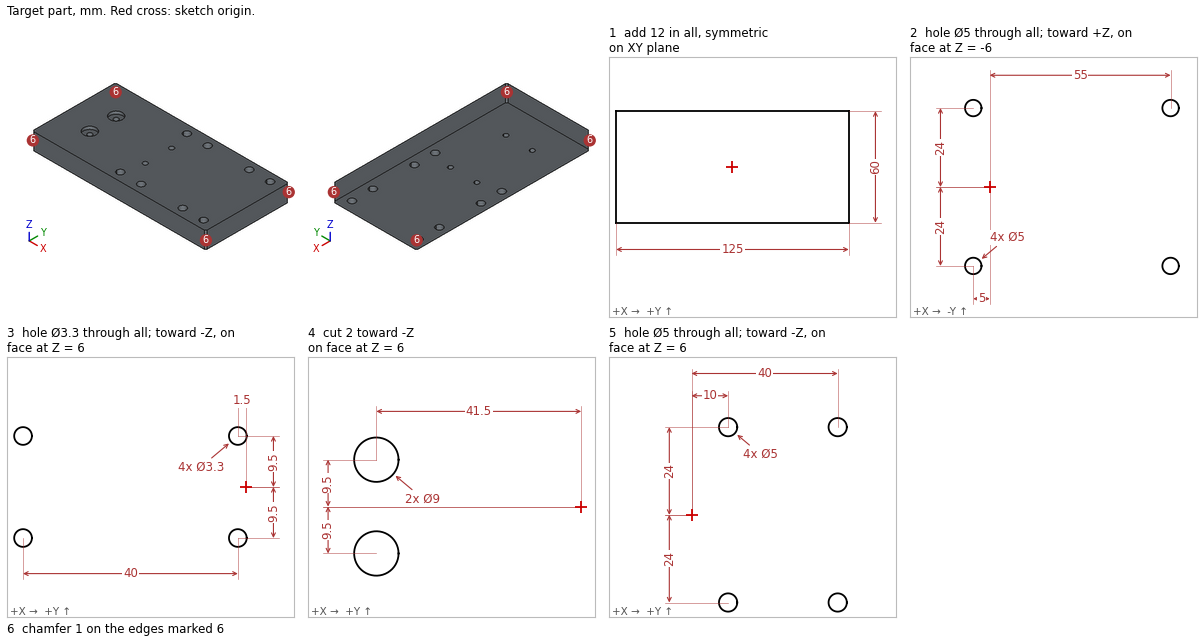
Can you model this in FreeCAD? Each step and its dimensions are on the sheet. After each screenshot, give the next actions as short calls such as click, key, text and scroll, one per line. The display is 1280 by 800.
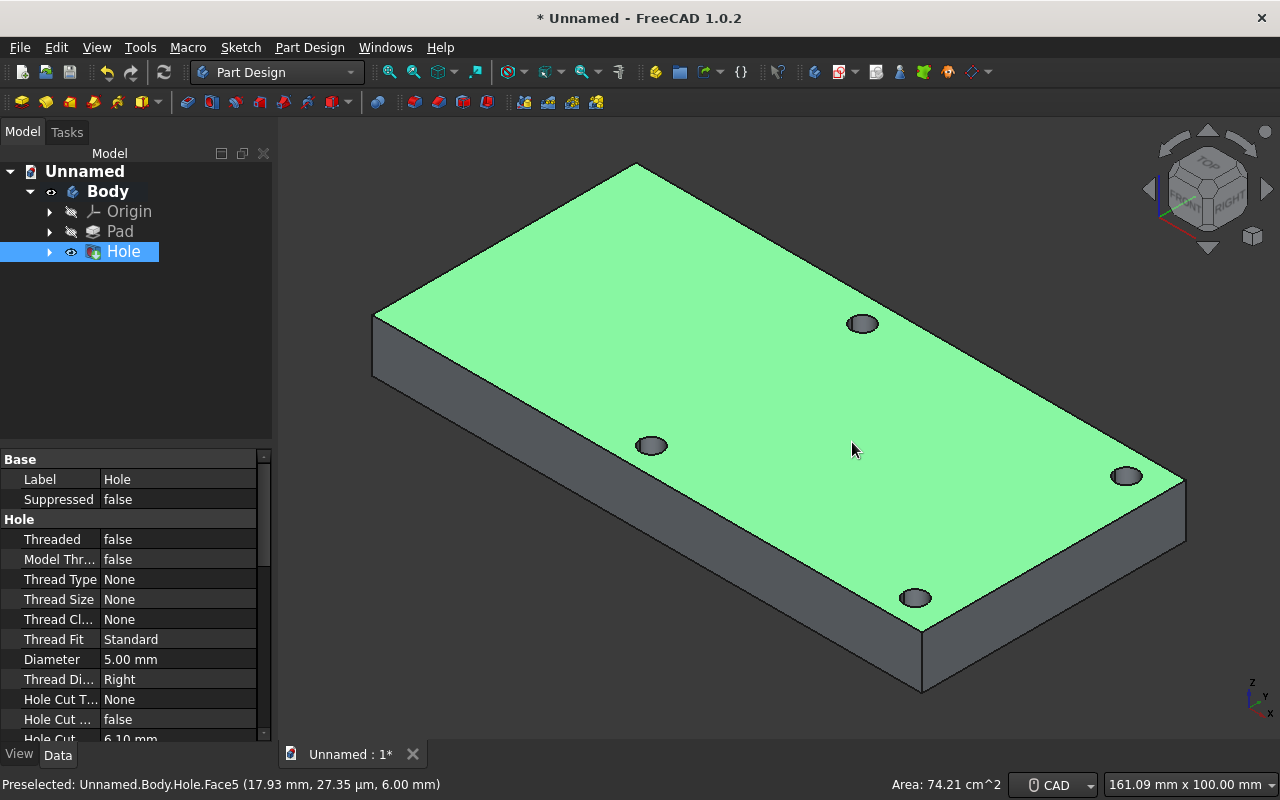
click(840, 72)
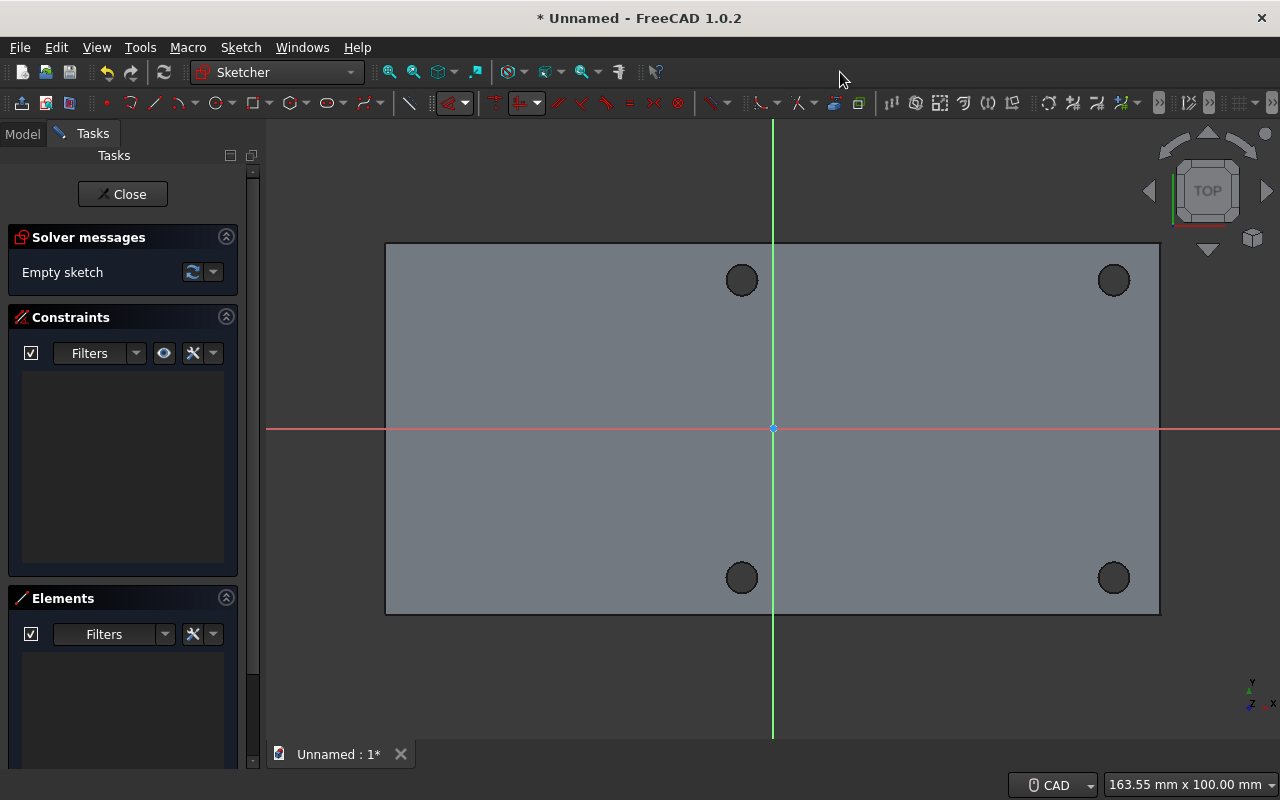
scroll(587, 429, up, 4)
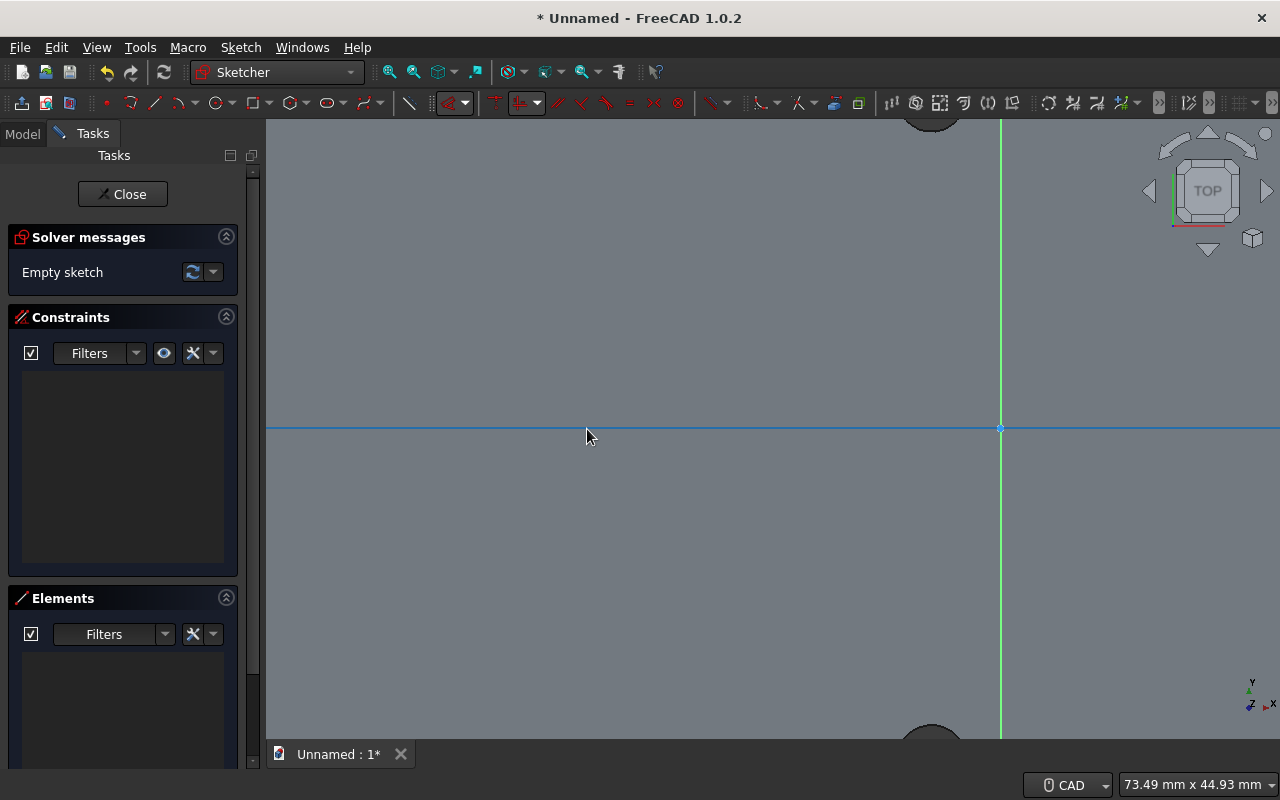
click(216, 104)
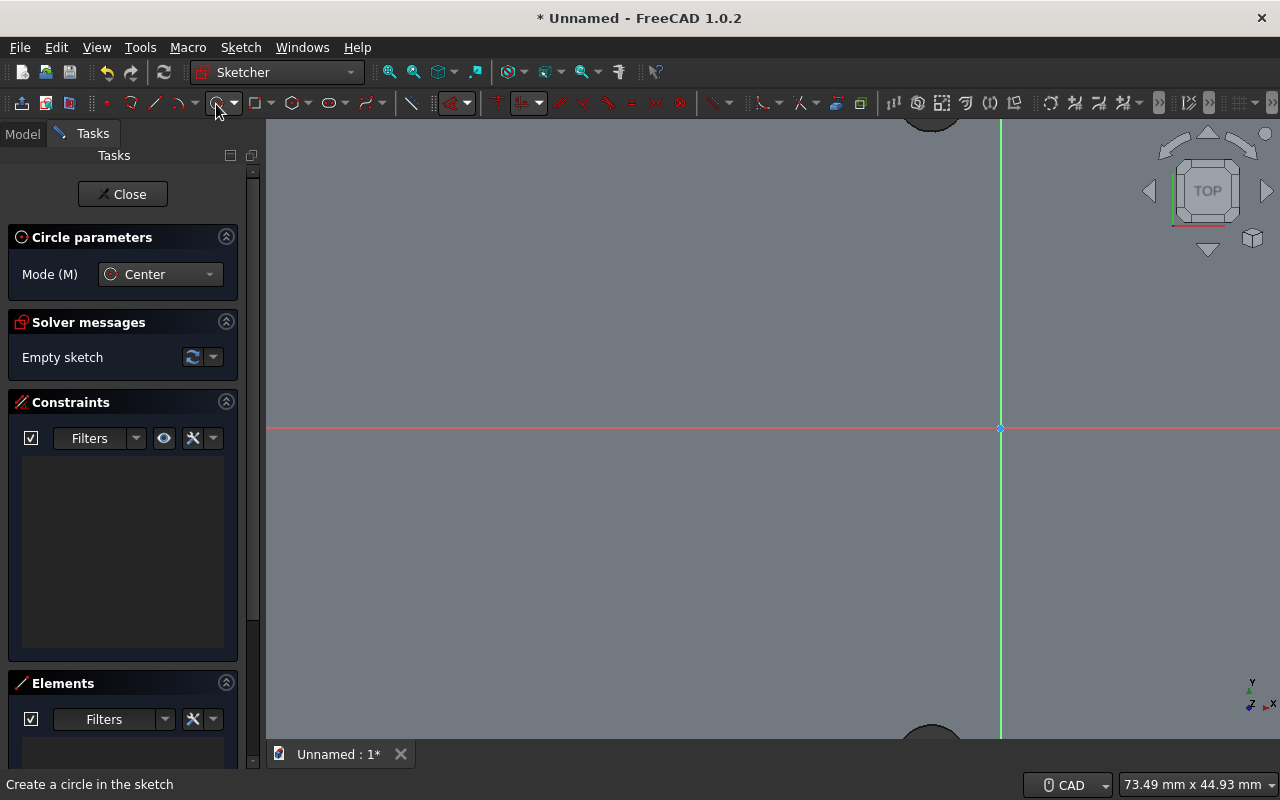
click(980, 297)
click(964, 281)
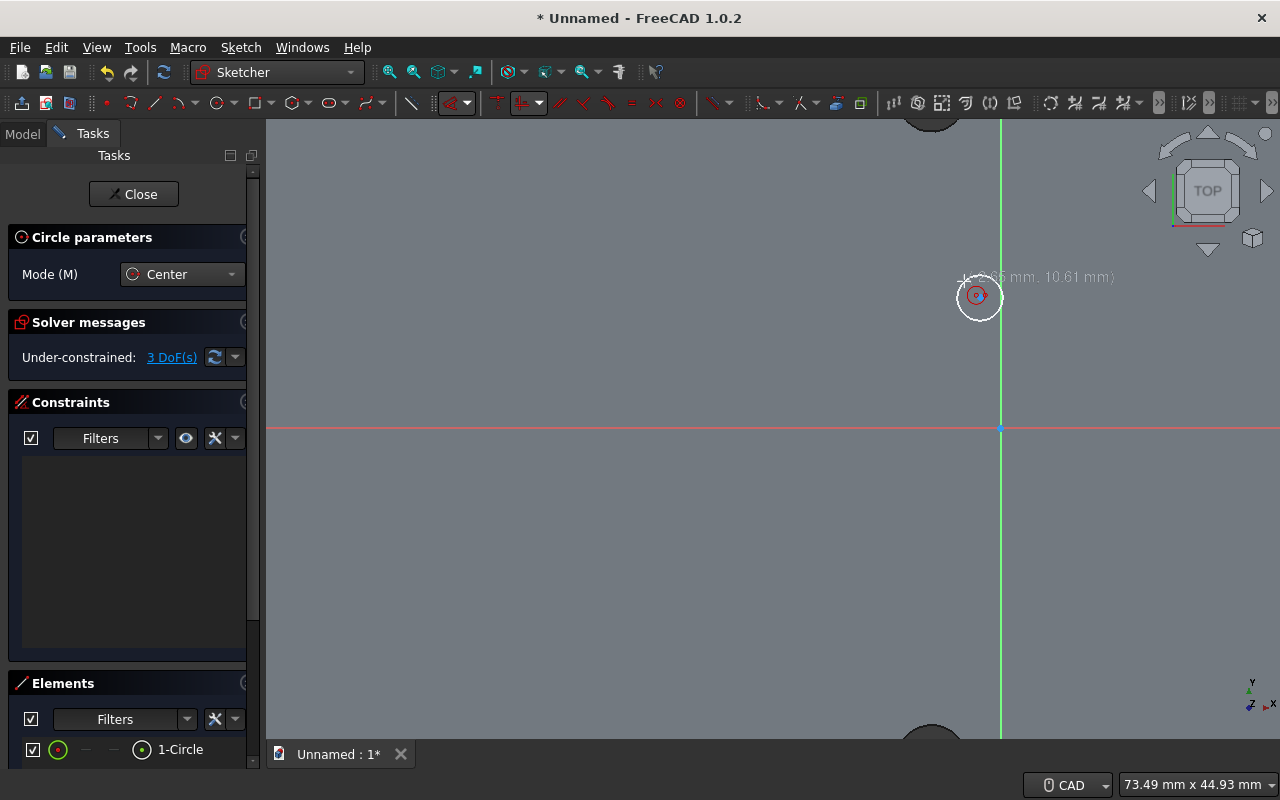
click(980, 559)
click(964, 543)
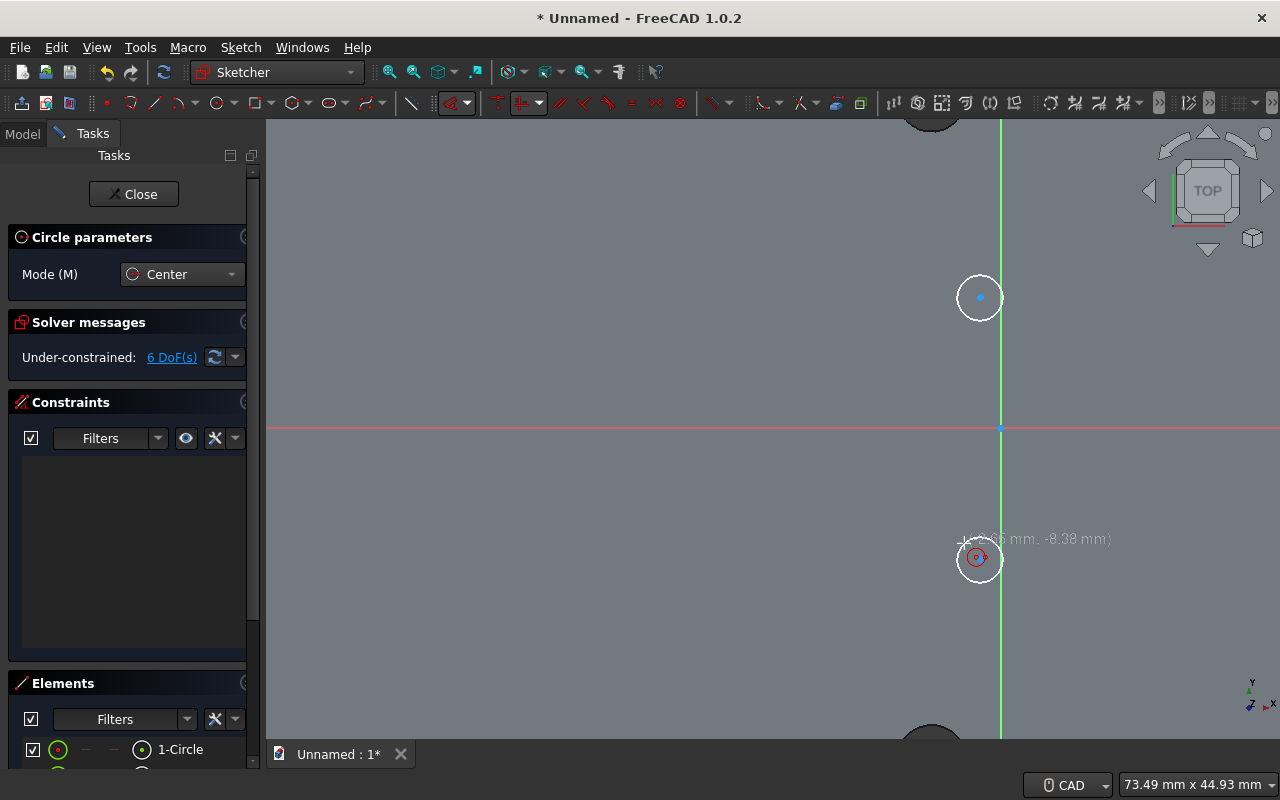
click(428, 559)
click(444, 543)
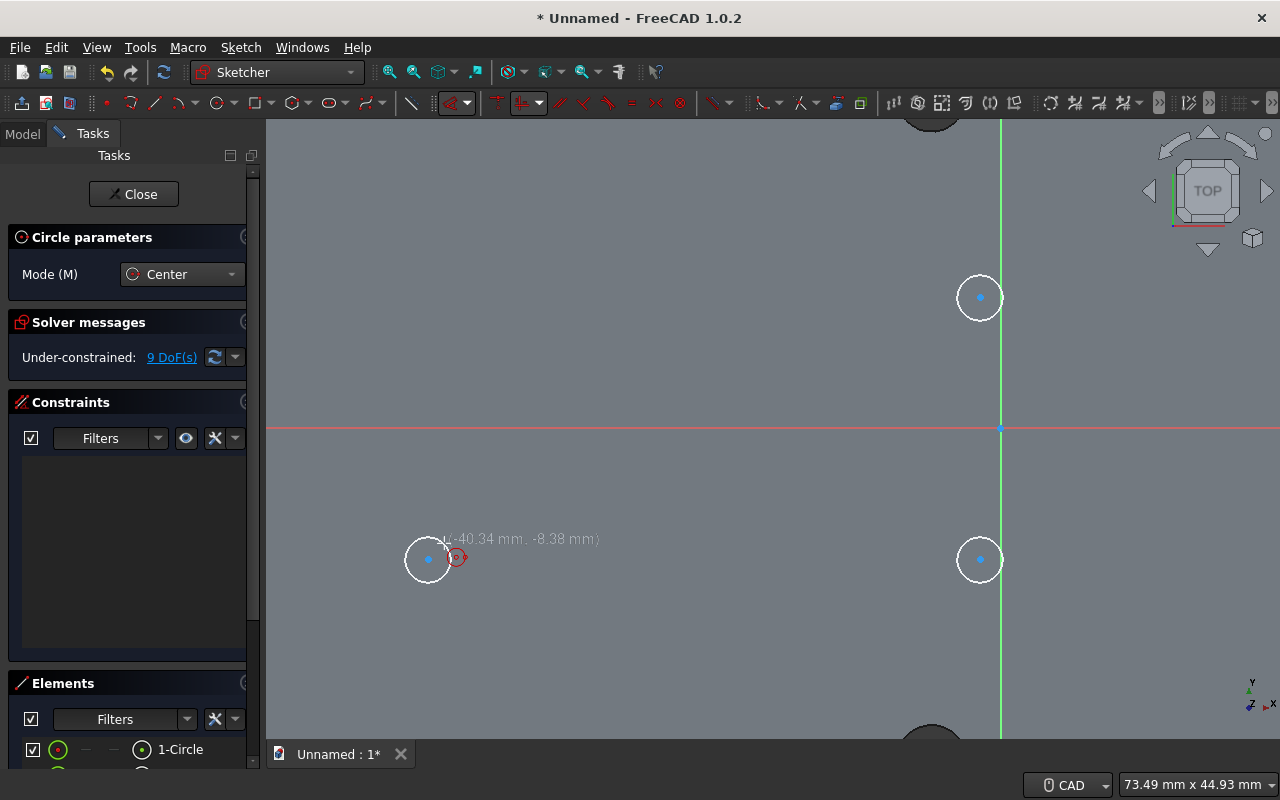
click(428, 297)
click(444, 281)
key(Escape)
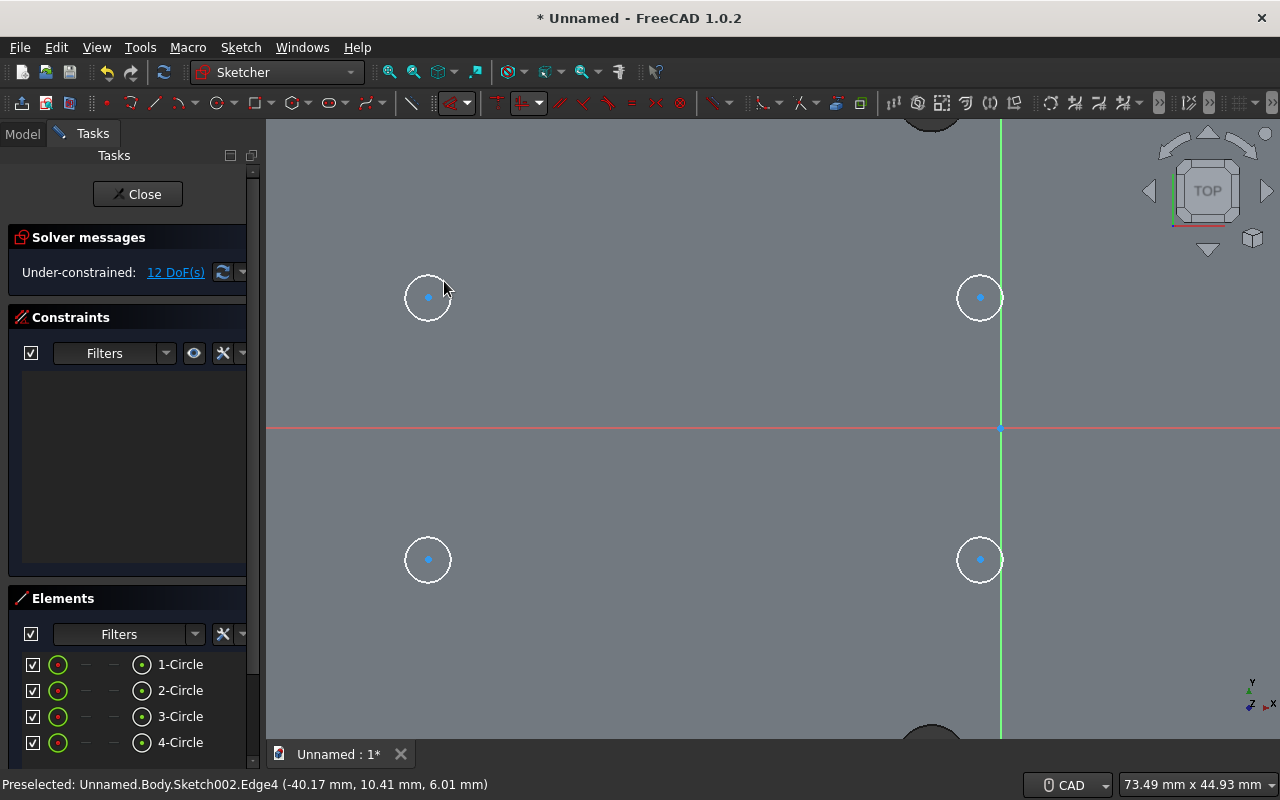
click(964, 282)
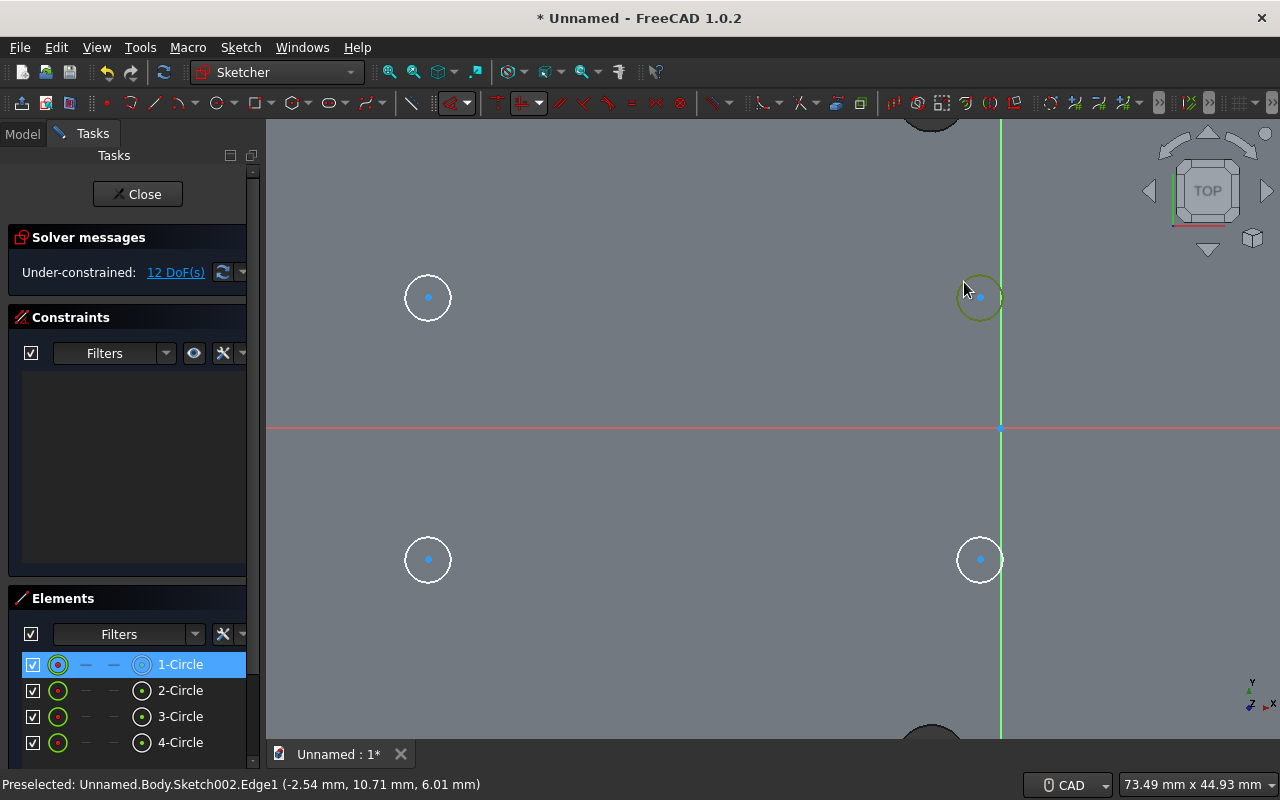
click(964, 544)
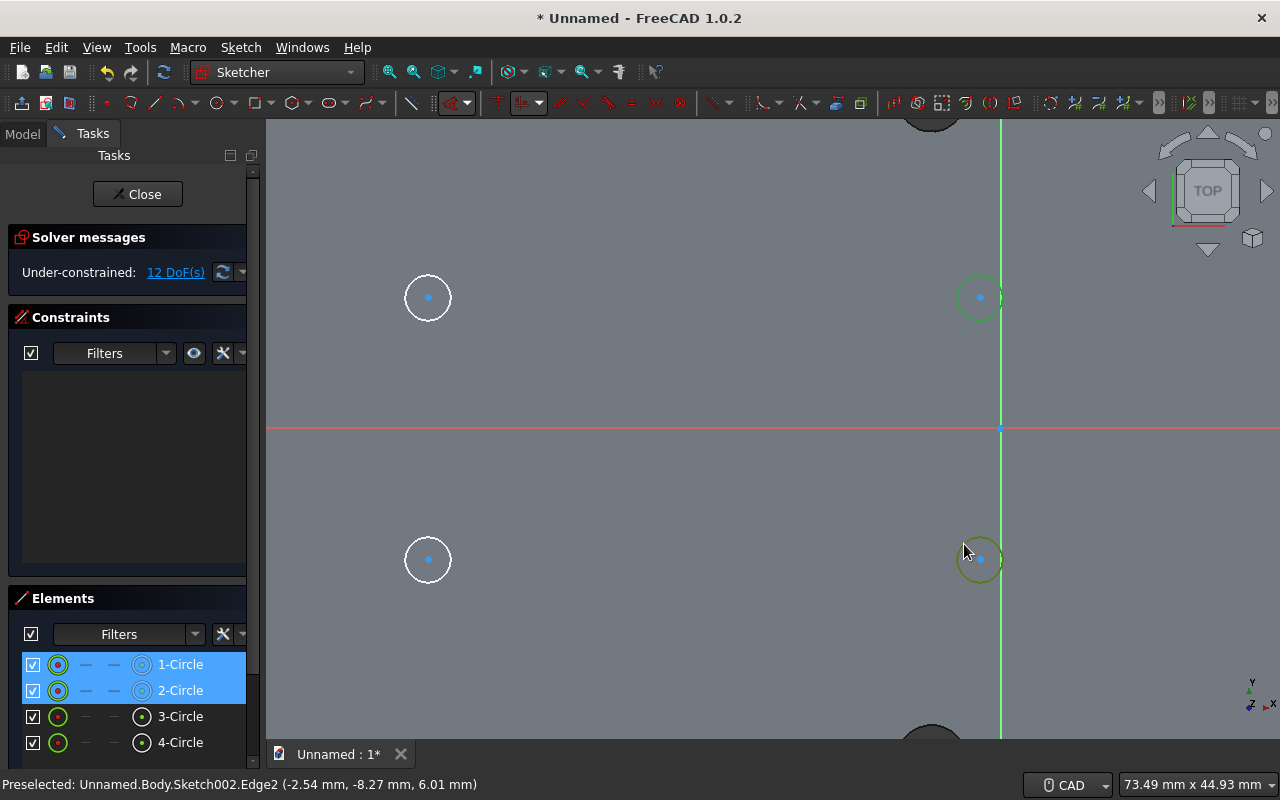
click(444, 544)